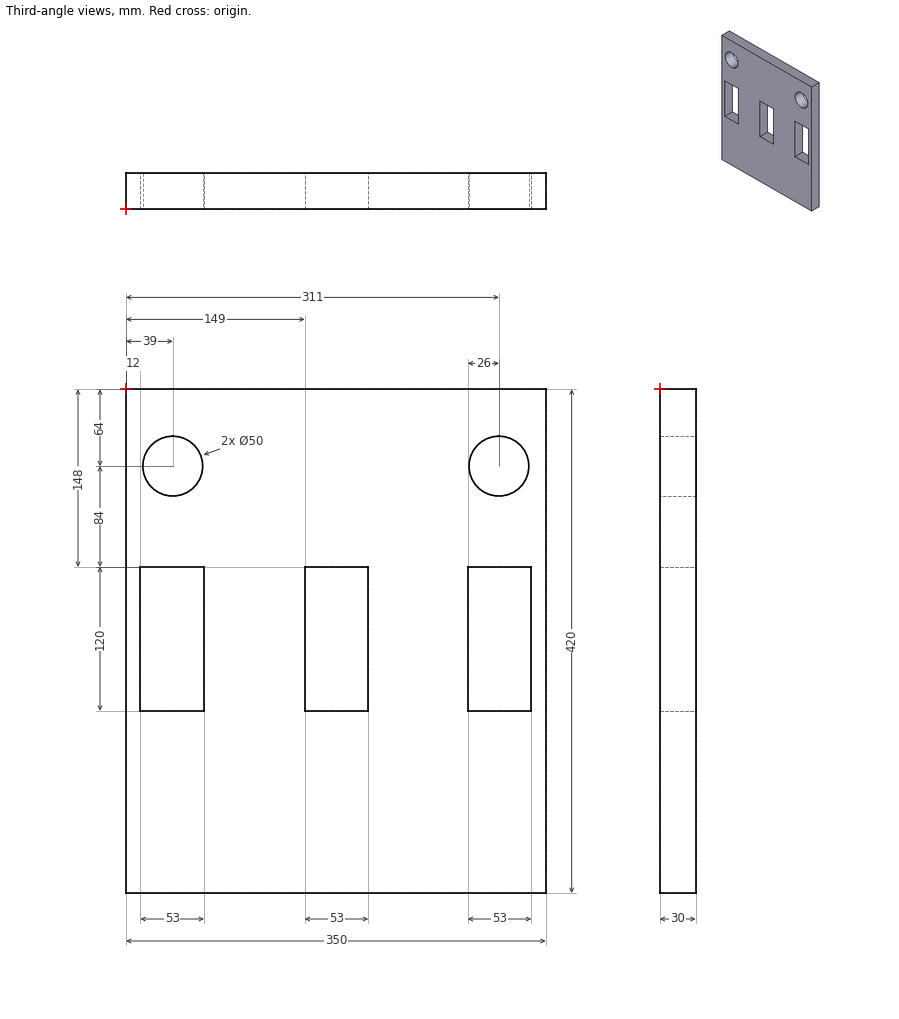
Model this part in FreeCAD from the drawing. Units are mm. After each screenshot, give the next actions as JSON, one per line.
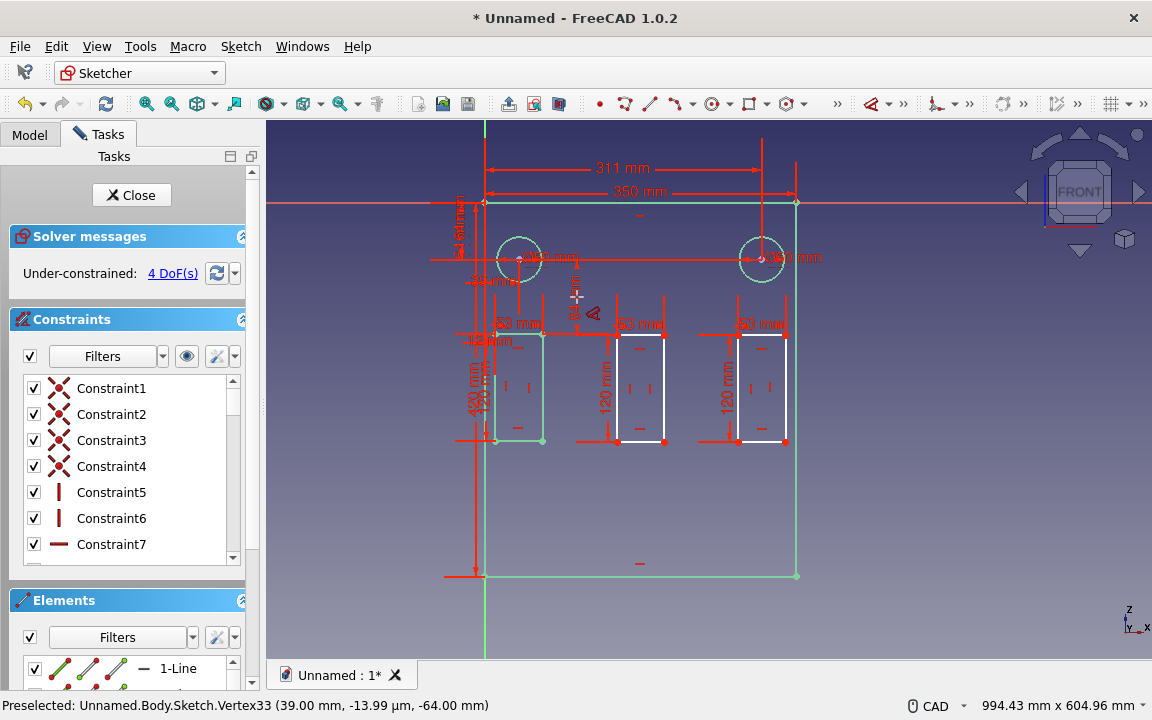
{"action": "scroll", "coordinate": [738, 335], "scroll_direction": "up", "scroll_amount": 3}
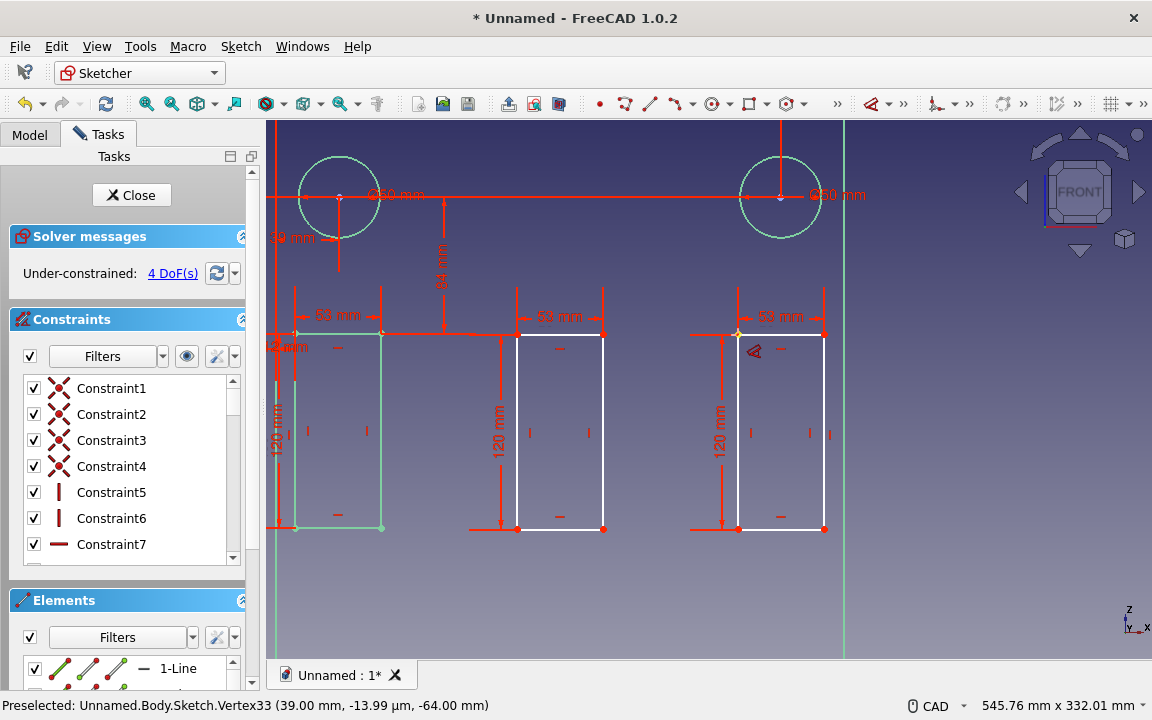
{"action": "left_click", "coordinate": [738, 335]}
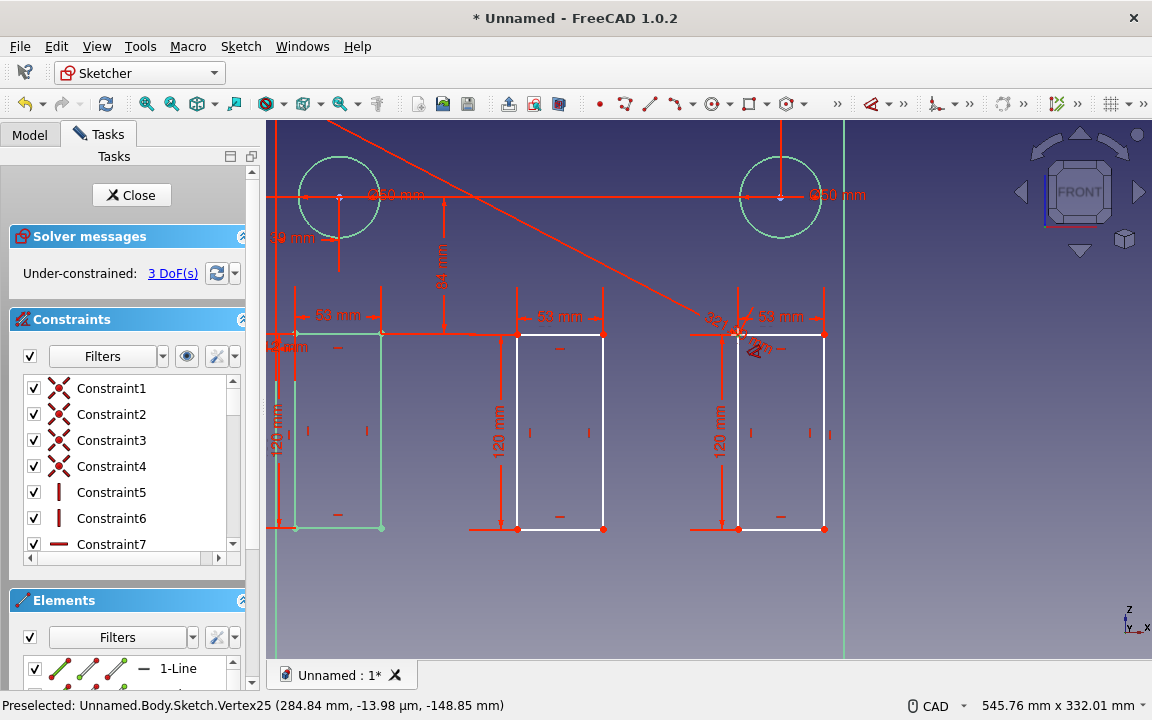
{"action": "left_click", "coordinate": [781, 197]}
{"action": "left_click", "coordinate": [760, 369]}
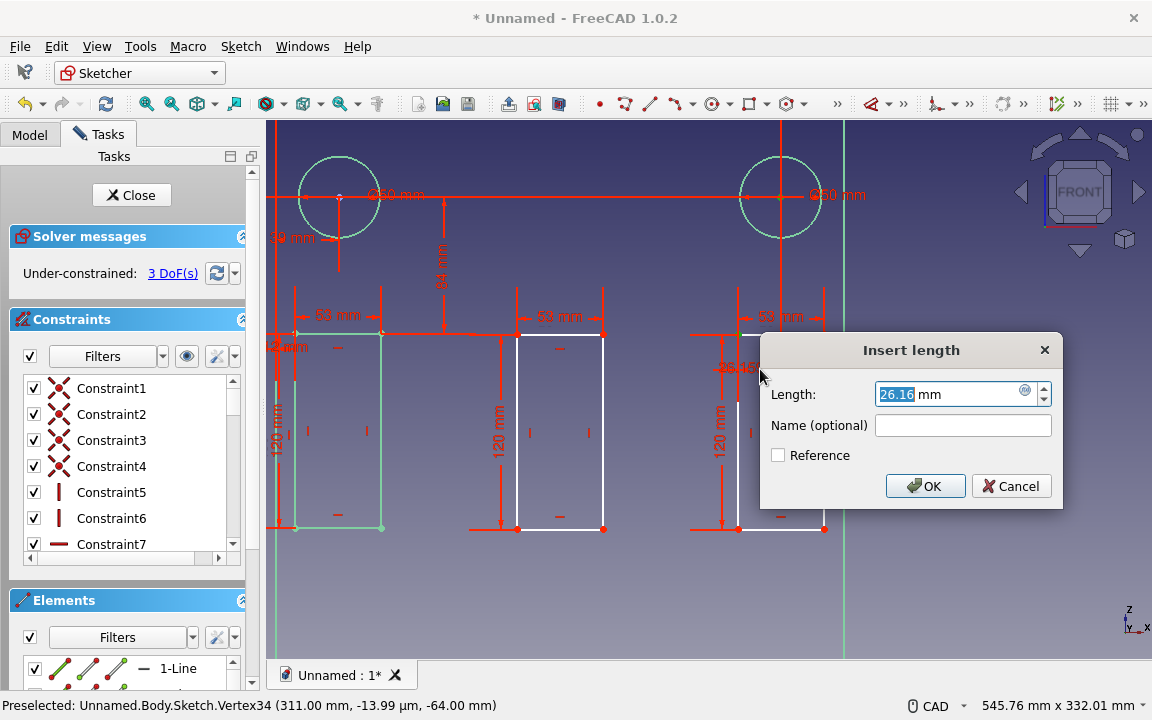
{"action": "type", "text": "26"}
{"action": "key", "text": "Return"}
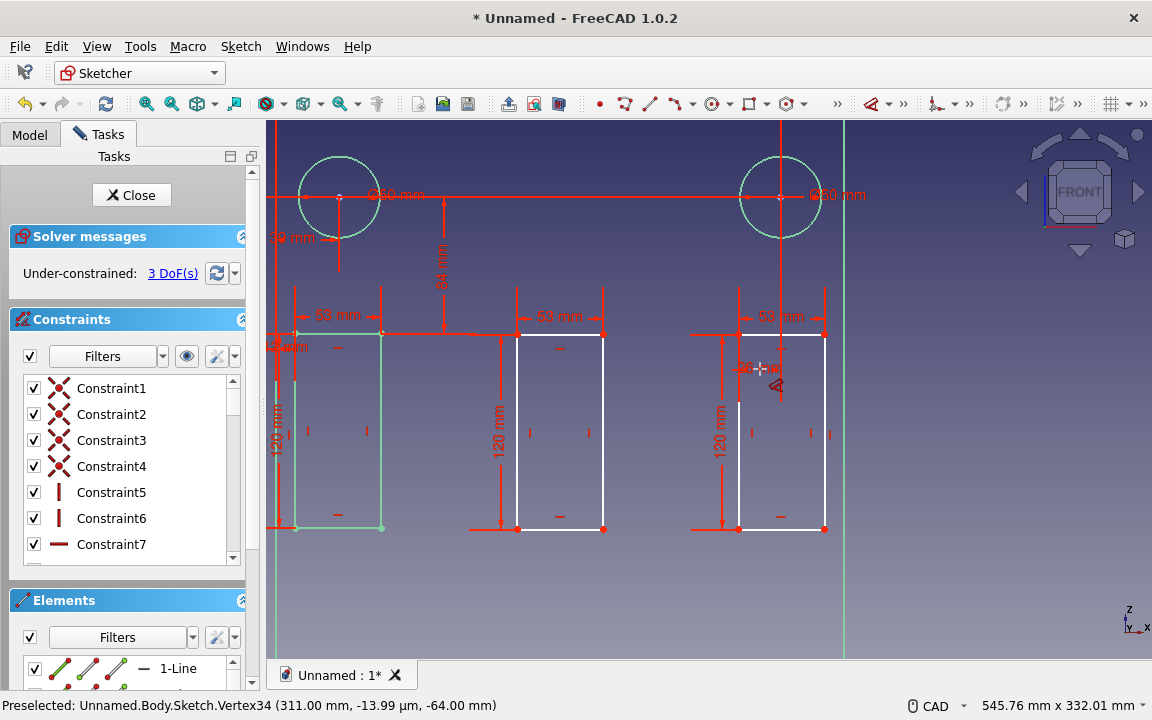
{"action": "left_click", "coordinate": [739, 335]}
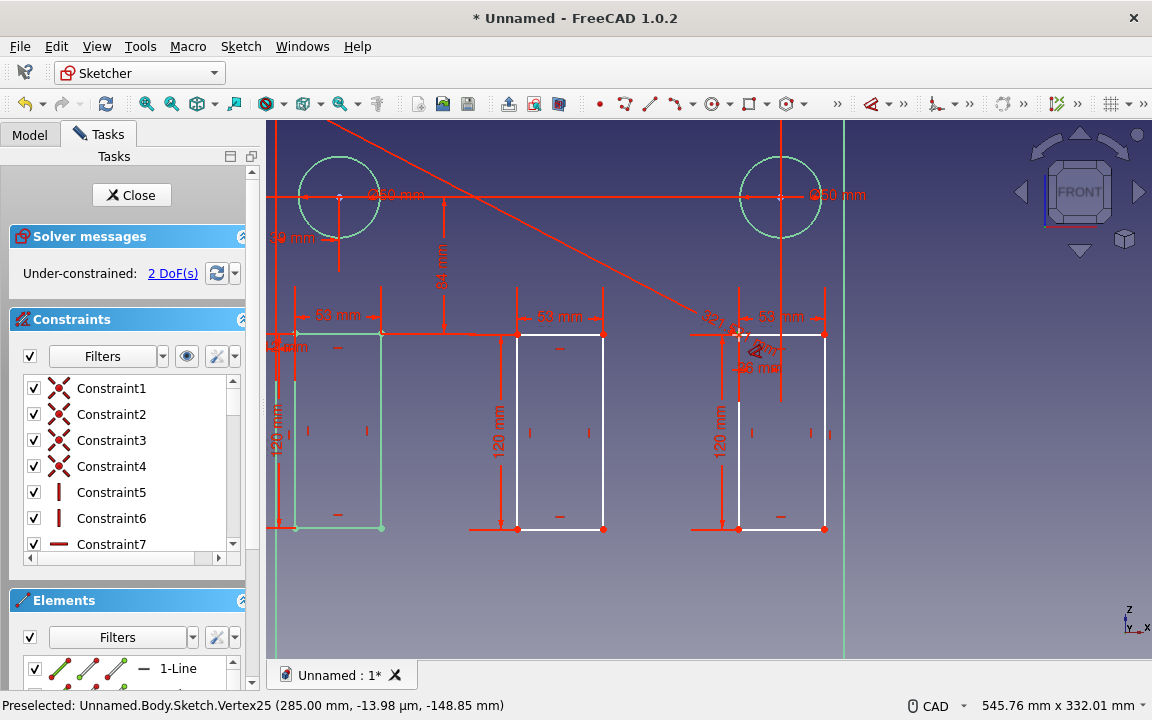
{"action": "left_click", "coordinate": [781, 197]}
{"action": "left_click", "coordinate": [815, 266]}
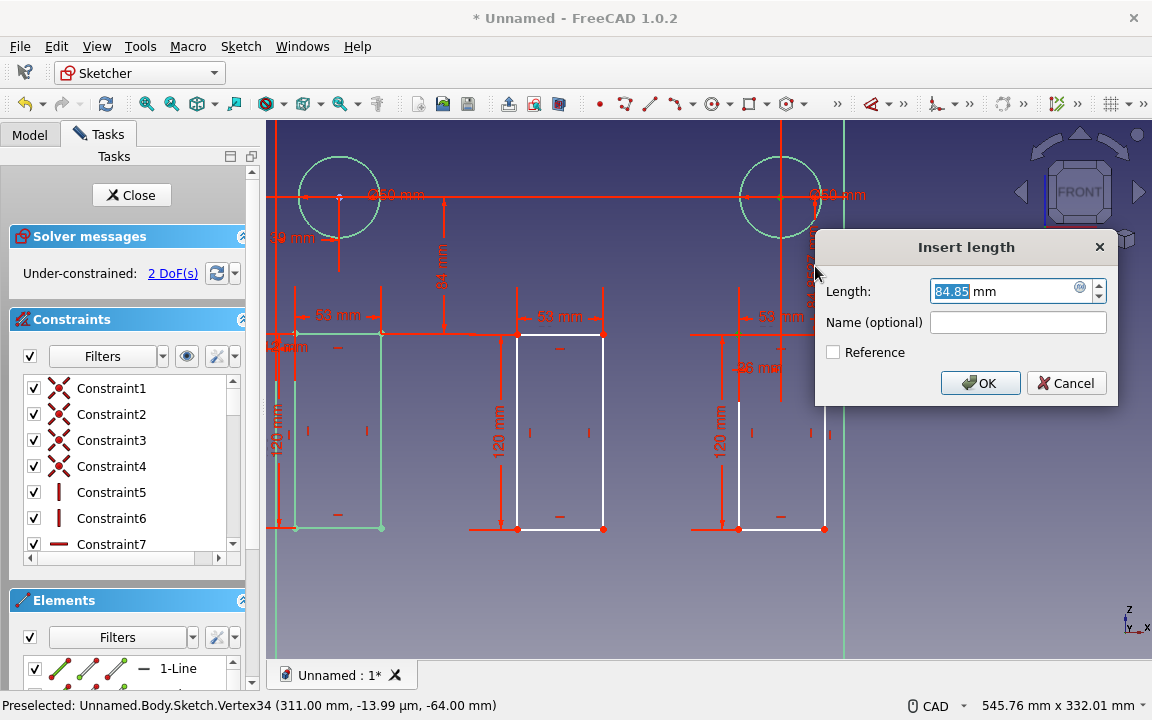
{"action": "type", "text": "84"}
{"action": "key", "text": "Return"}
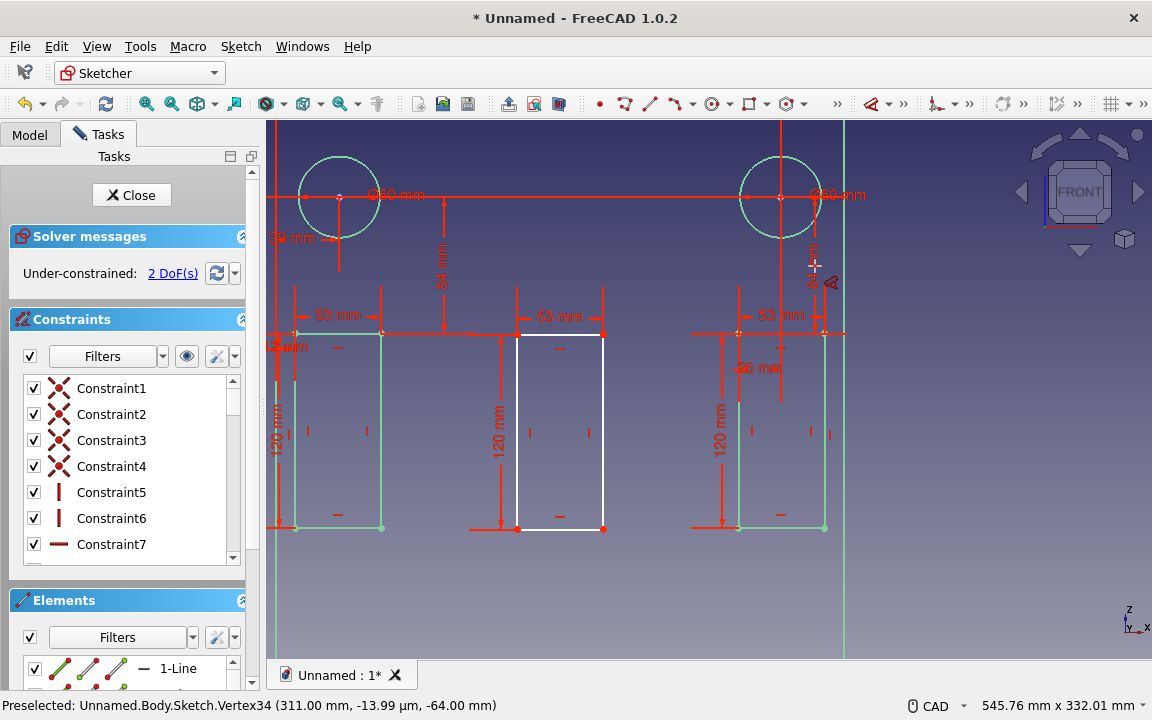
{"action": "left_click", "coordinate": [517, 335]}
{"action": "left_click", "coordinate": [406, 369]}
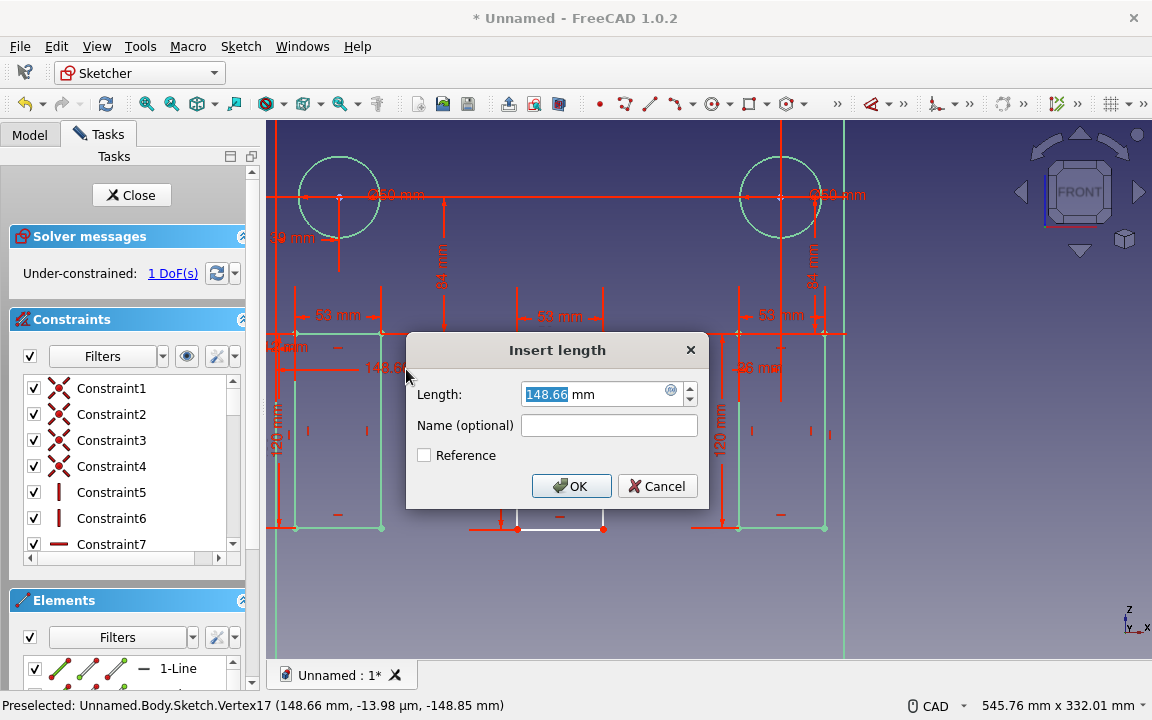
{"action": "type", "text": "149"}
{"action": "key", "text": "Return"}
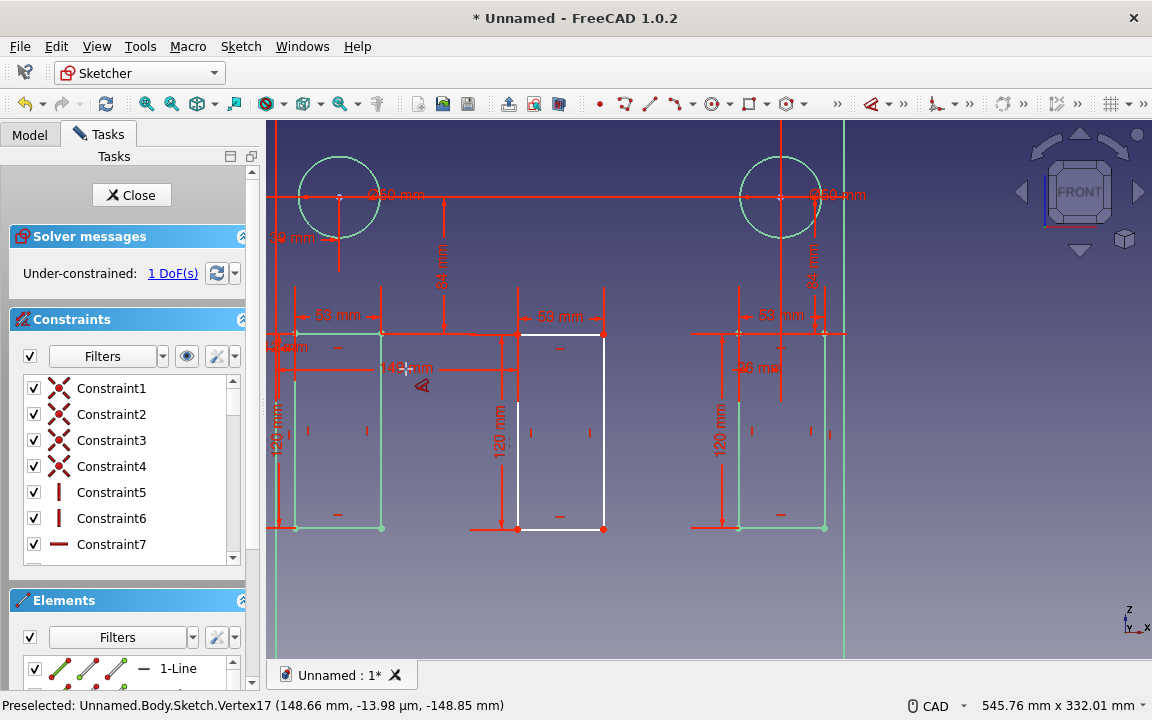
{"action": "left_click", "coordinate": [518, 335]}
{"action": "left_click", "coordinate": [552, 241]}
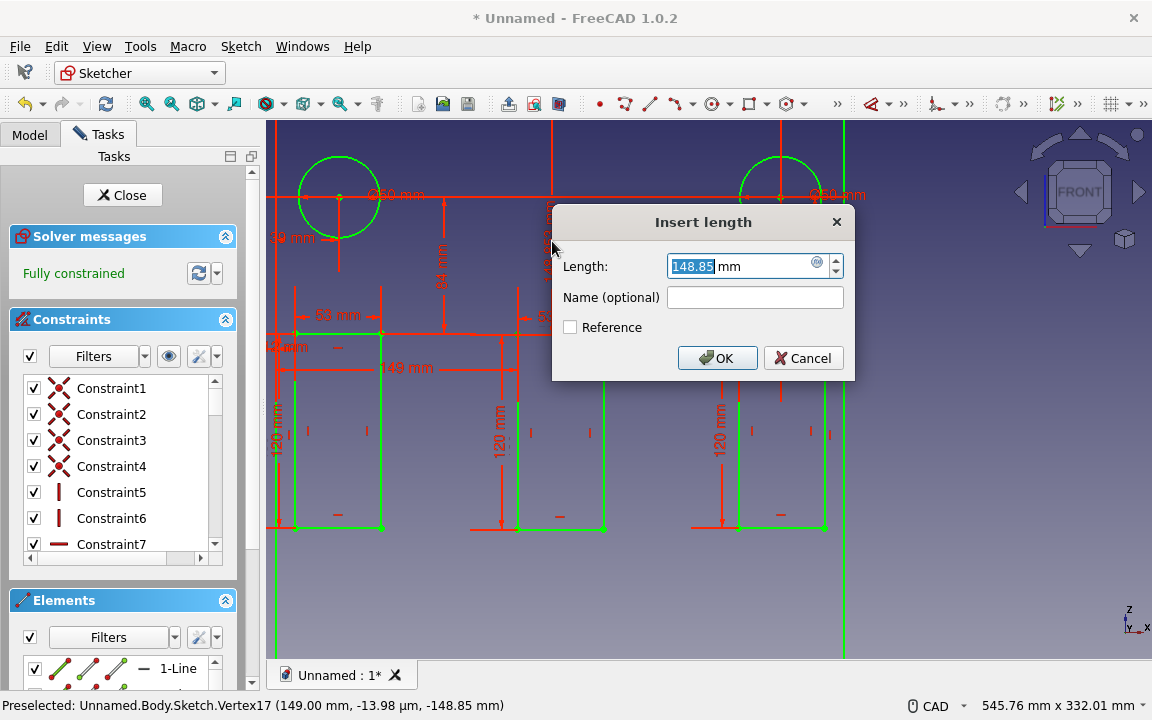
{"action": "type", "text": "148"}
{"action": "key", "text": "Return"}
{"action": "key", "text": "Escape"}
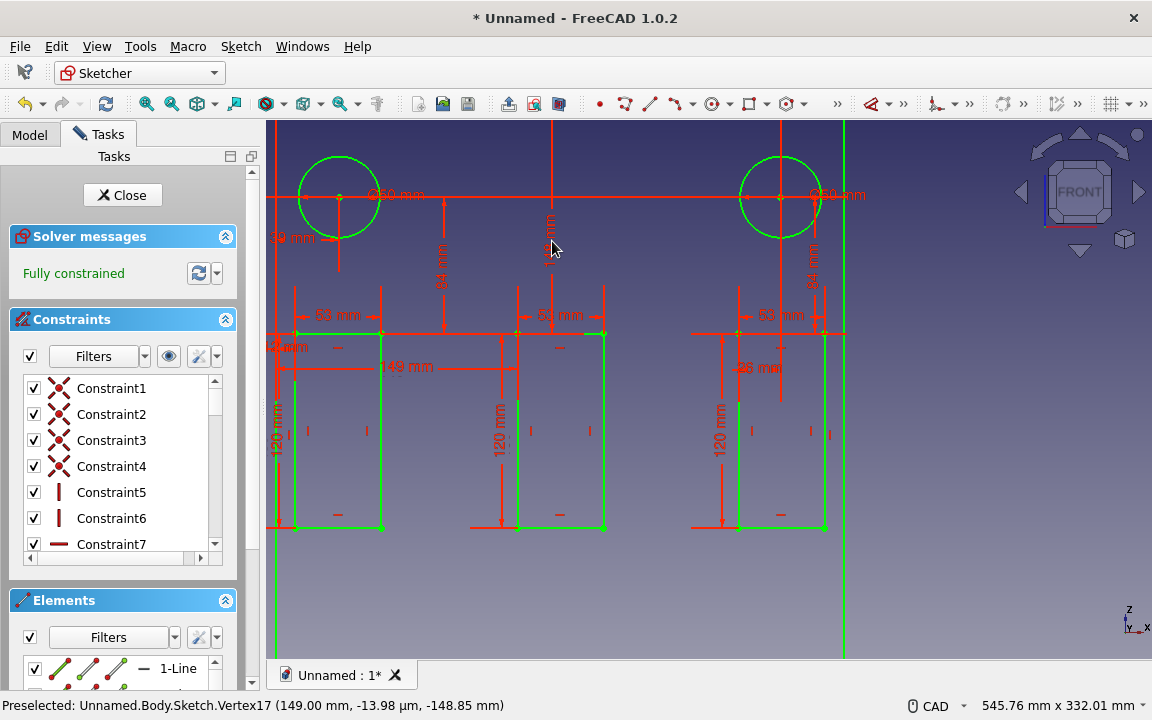
{"action": "left_click", "coordinate": [123, 195]}